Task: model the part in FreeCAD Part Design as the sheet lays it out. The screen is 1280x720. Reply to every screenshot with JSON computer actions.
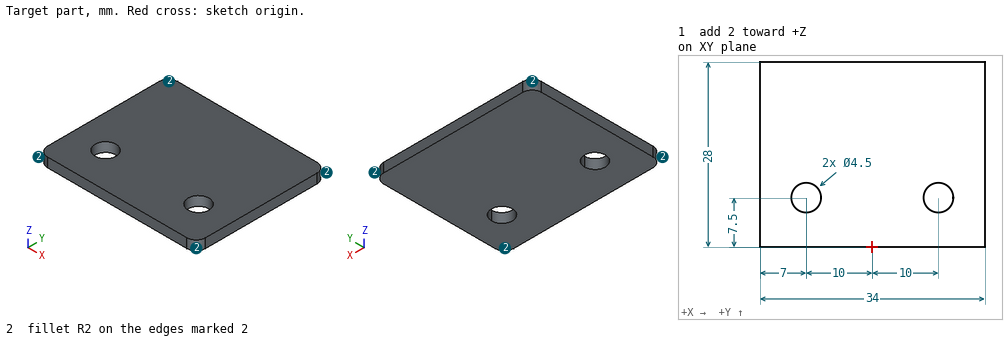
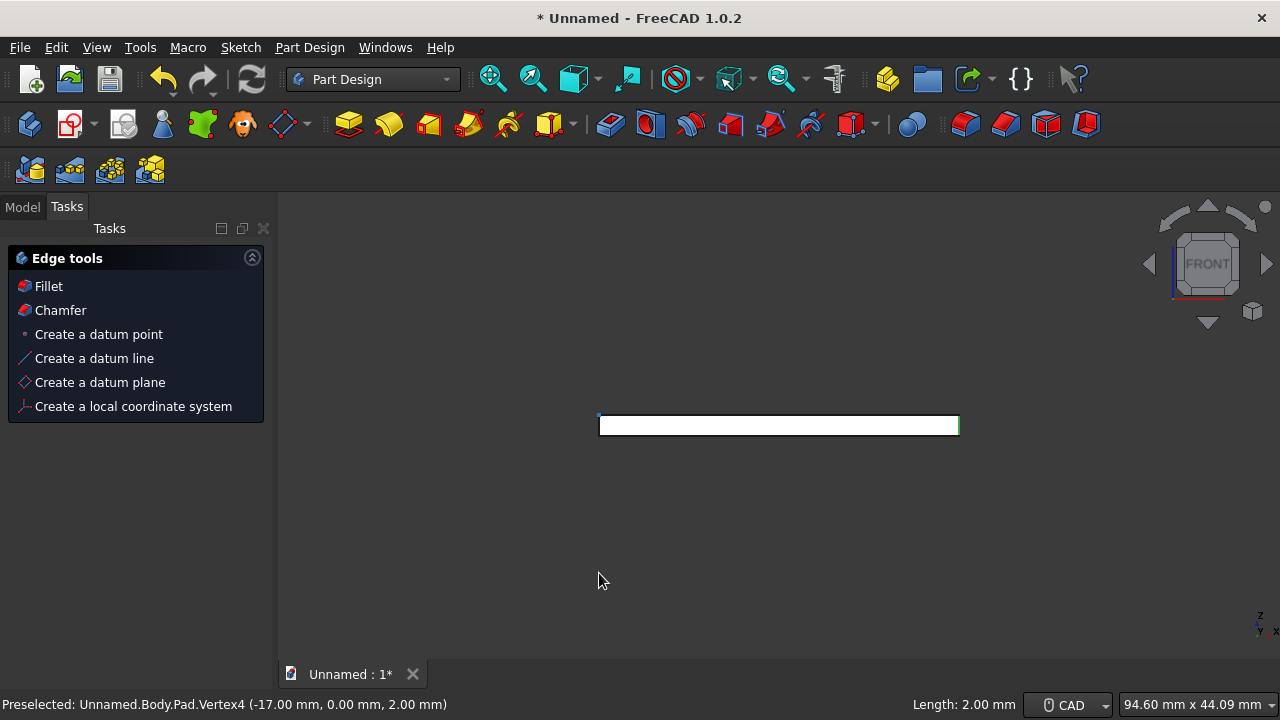
{"action": "left_click", "coordinate": [599, 425], "text": "ctrl"}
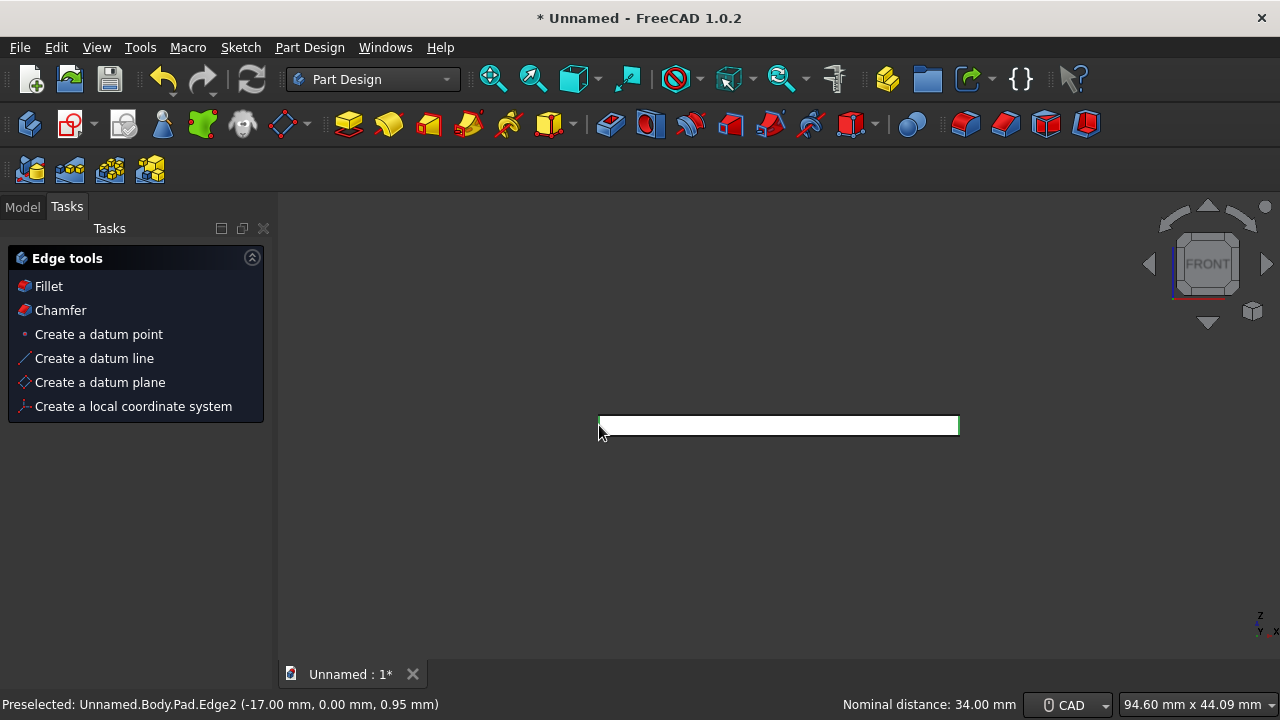
{"action": "scroll", "coordinate": [599, 425], "scroll_direction": "up", "scroll_amount": 4}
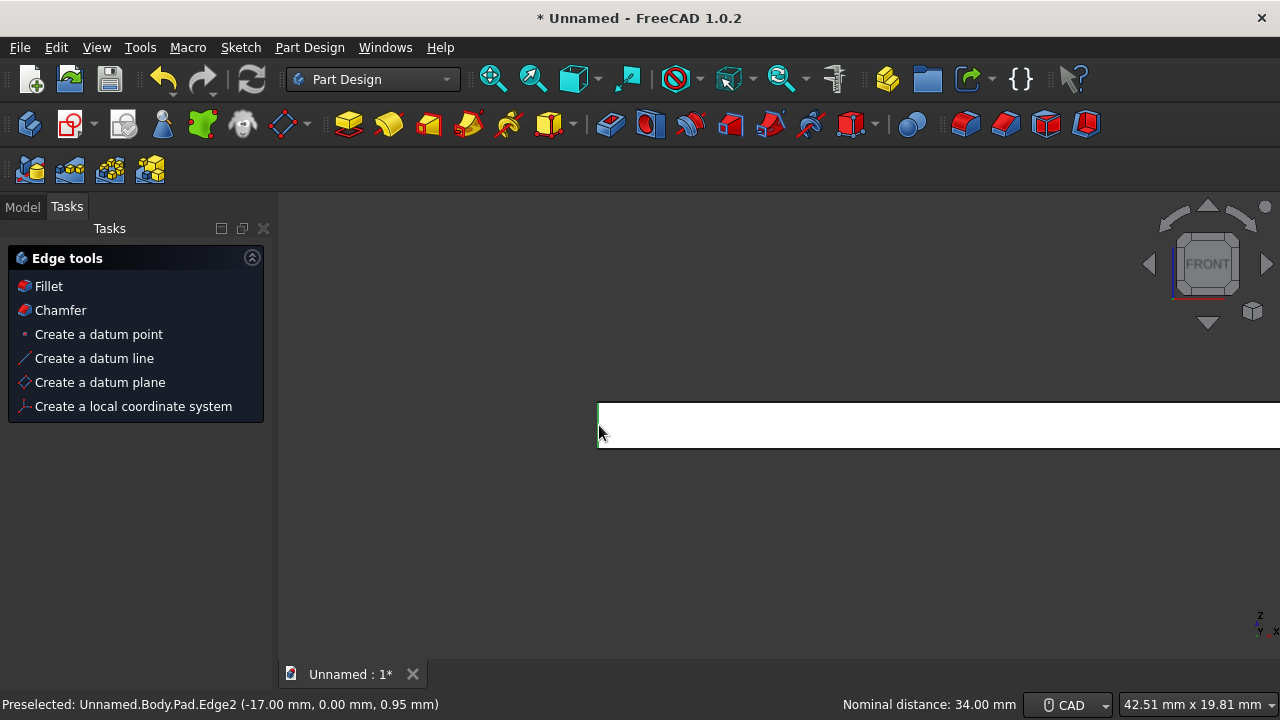
{"action": "key", "text": "v f"}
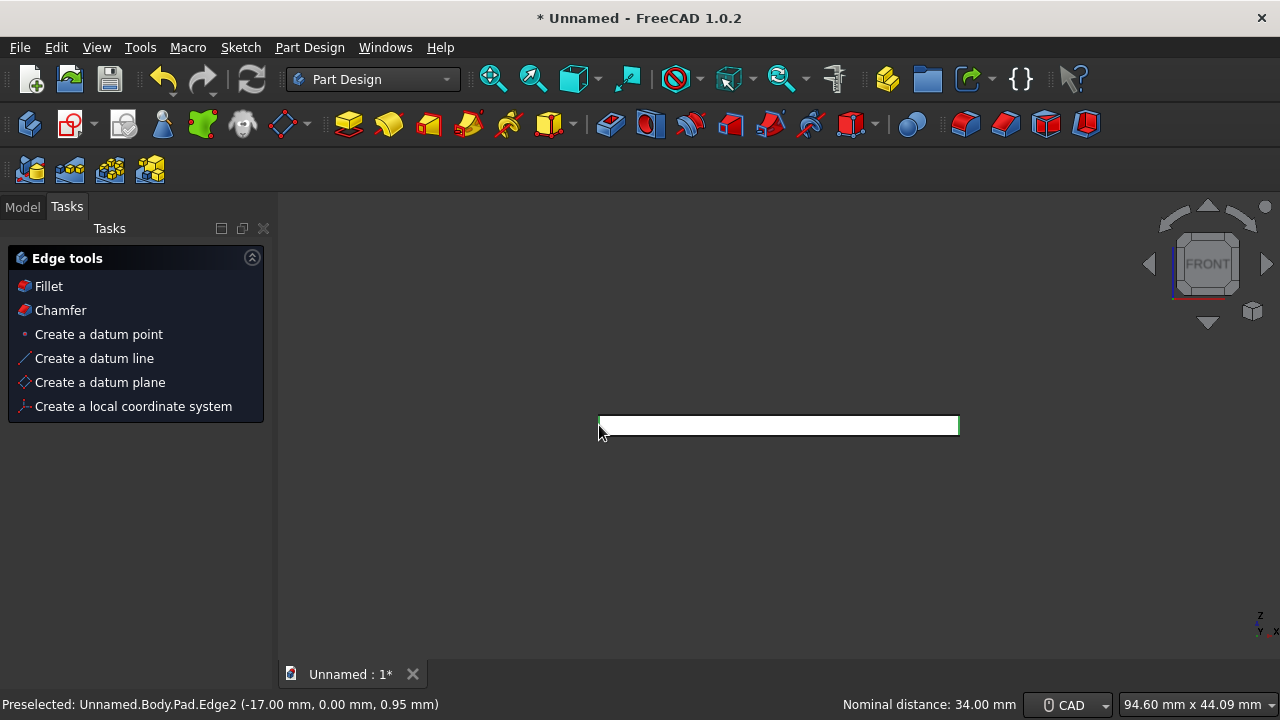
{"action": "key", "text": "3"}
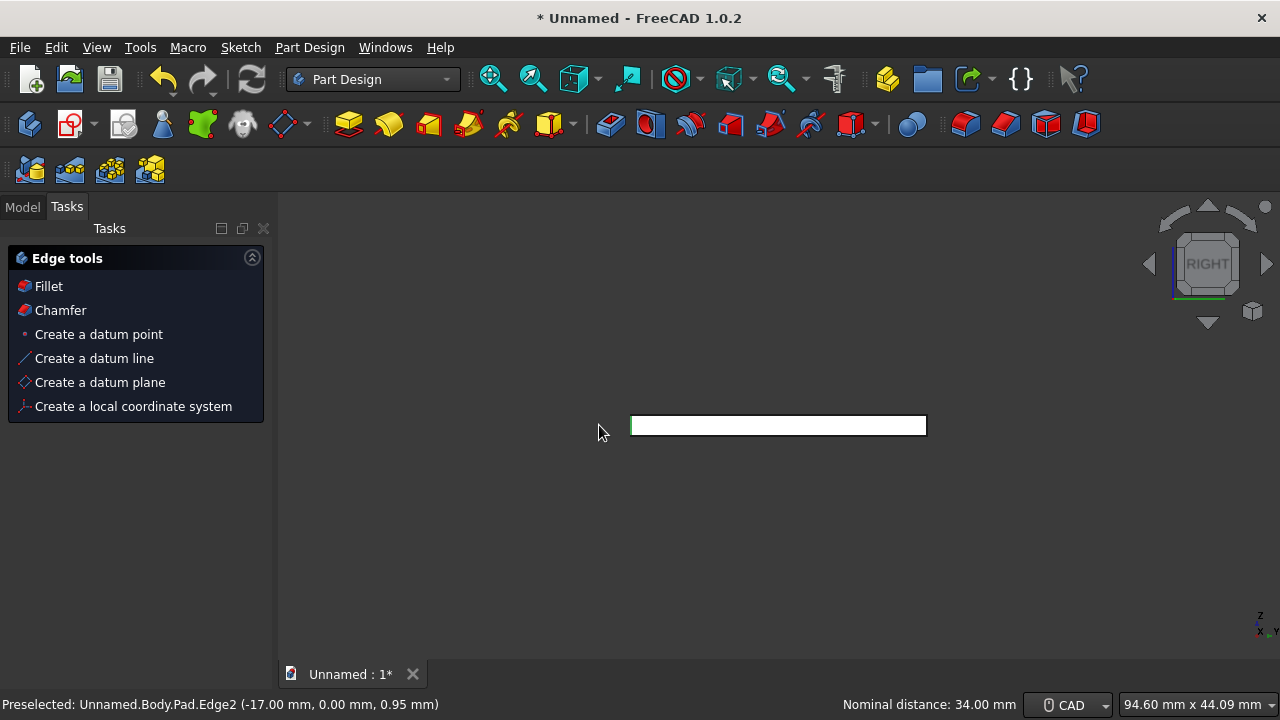
{"action": "left_click", "coordinate": [494, 80]}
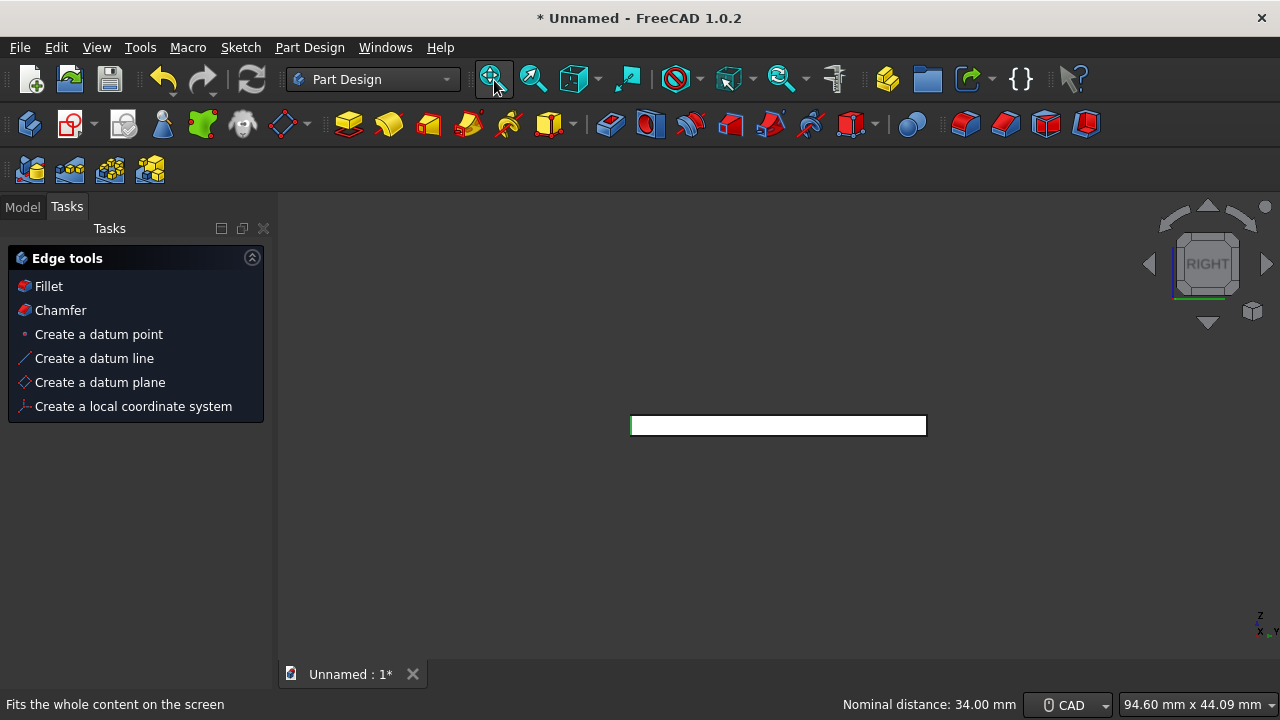
{"action": "left_click", "coordinate": [927, 424], "text": "ctrl"}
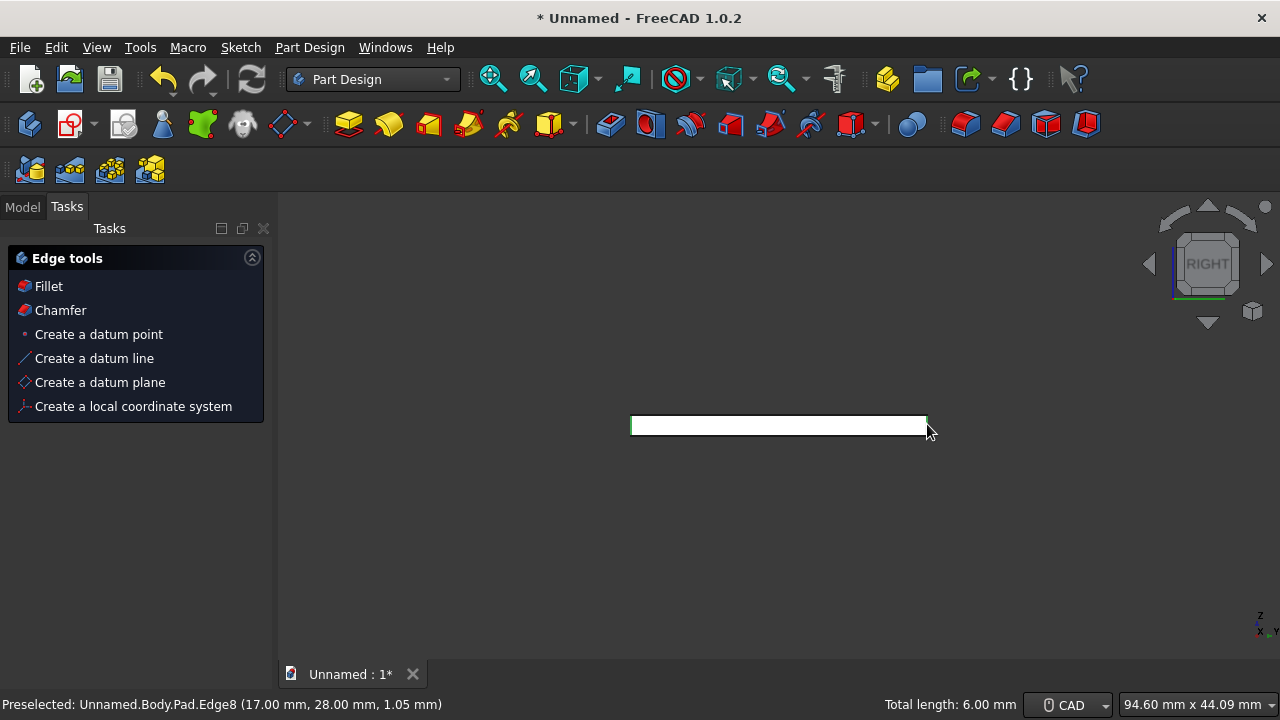
{"action": "scroll", "coordinate": [927, 424], "scroll_direction": "up", "scroll_amount": 4}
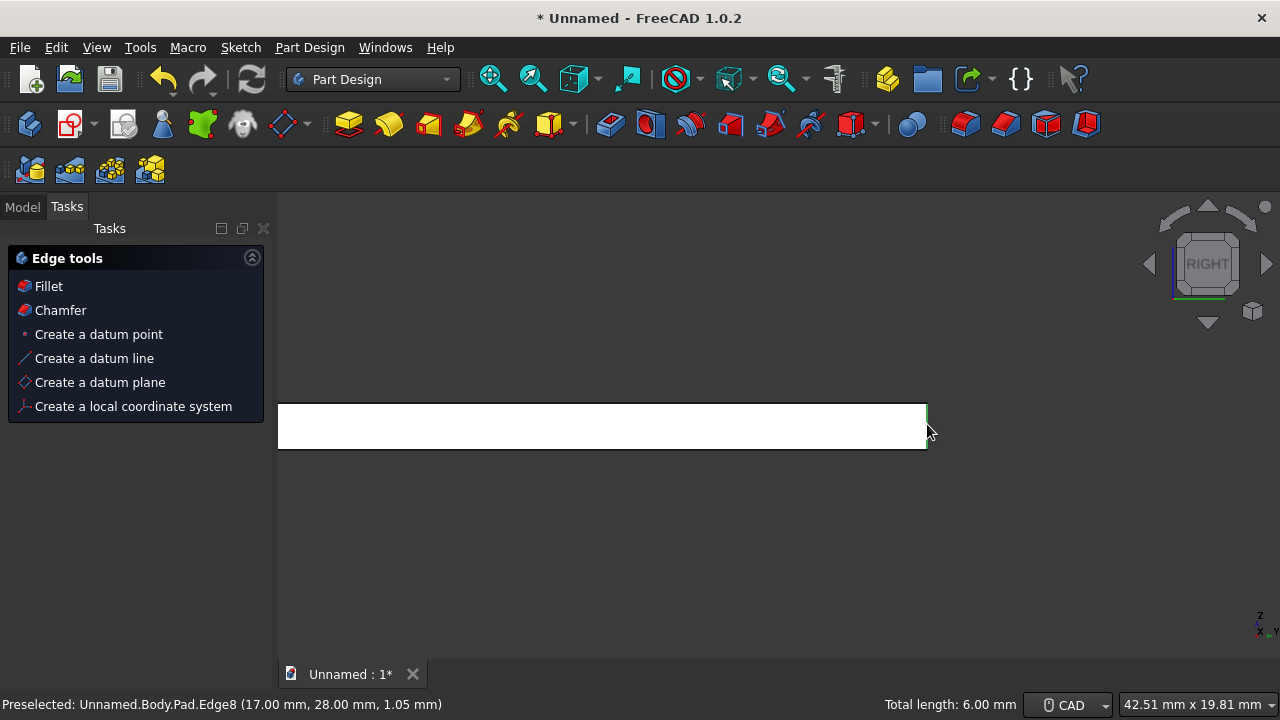
{"action": "key", "text": "v f"}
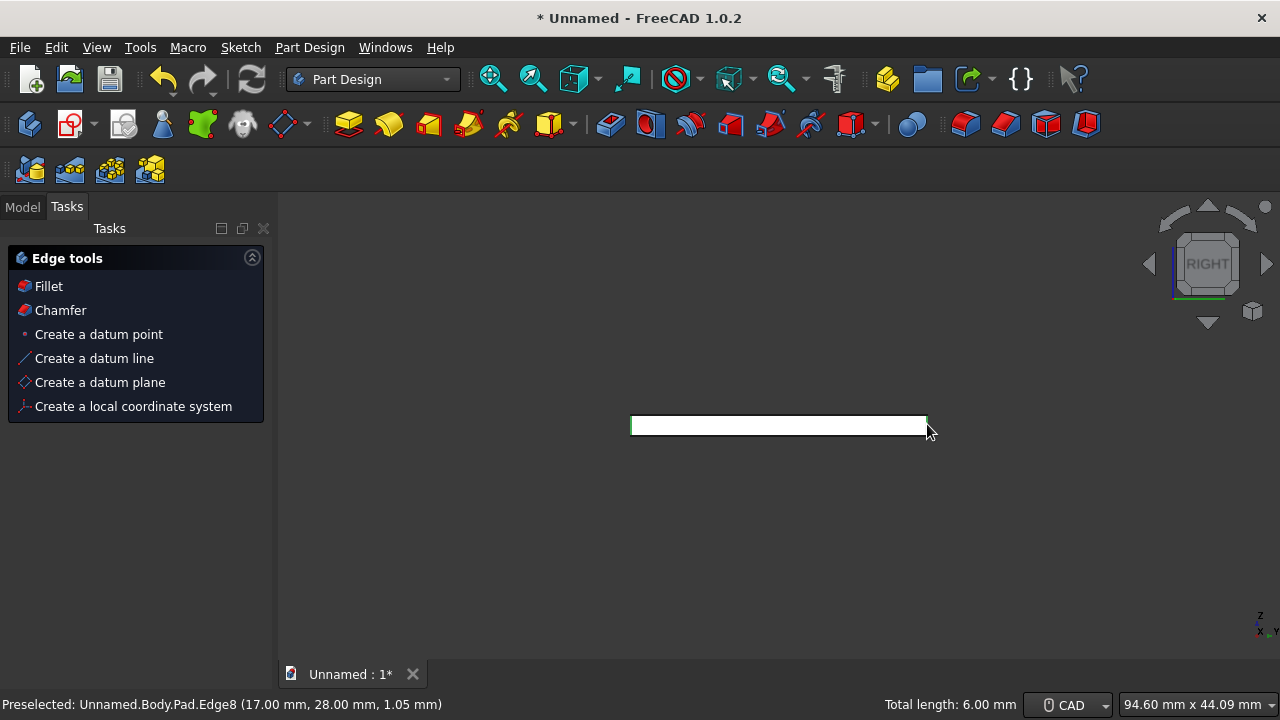
{"action": "key", "text": "5"}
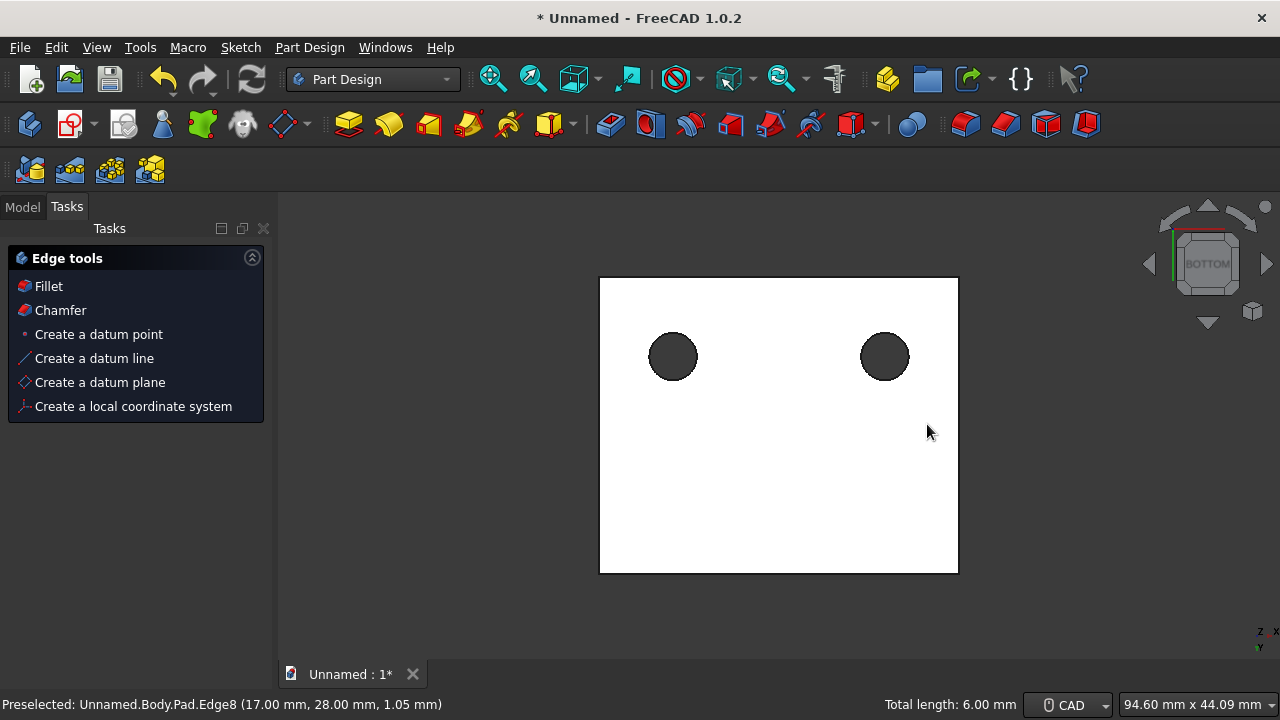
{"action": "scroll", "coordinate": [599, 573], "scroll_direction": "up", "scroll_amount": 4}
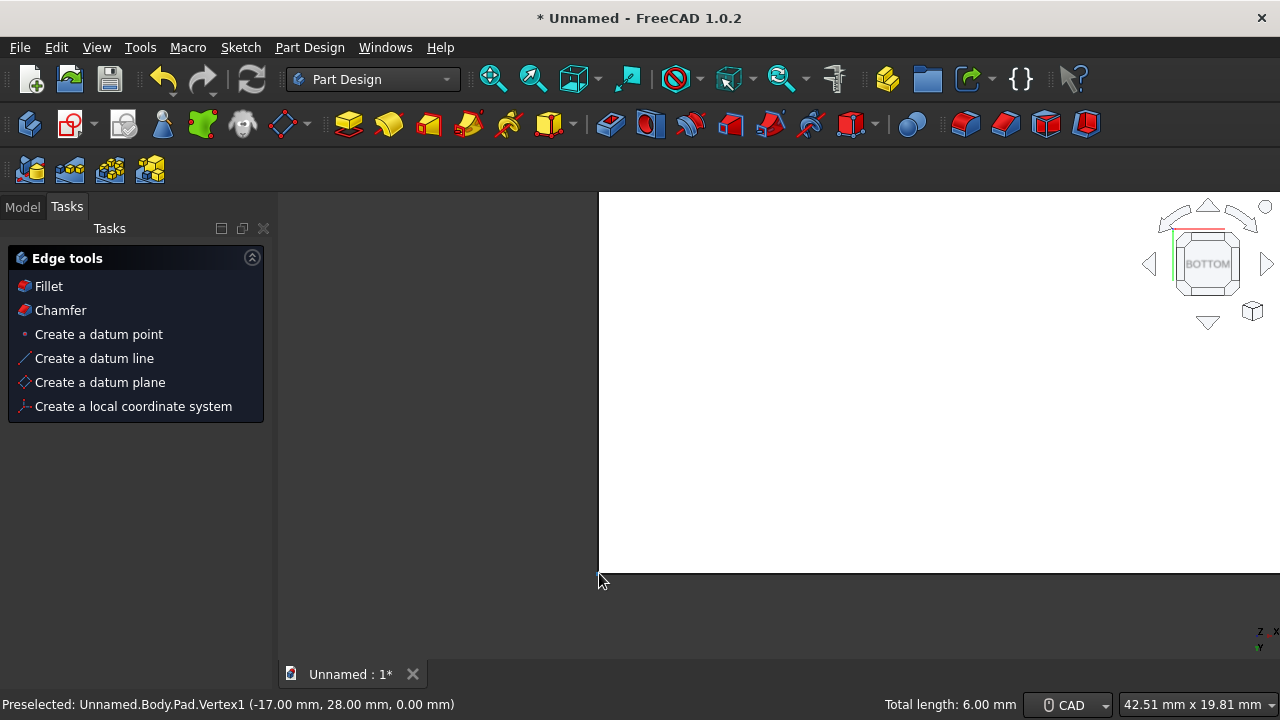
{"action": "key", "text": "v f"}